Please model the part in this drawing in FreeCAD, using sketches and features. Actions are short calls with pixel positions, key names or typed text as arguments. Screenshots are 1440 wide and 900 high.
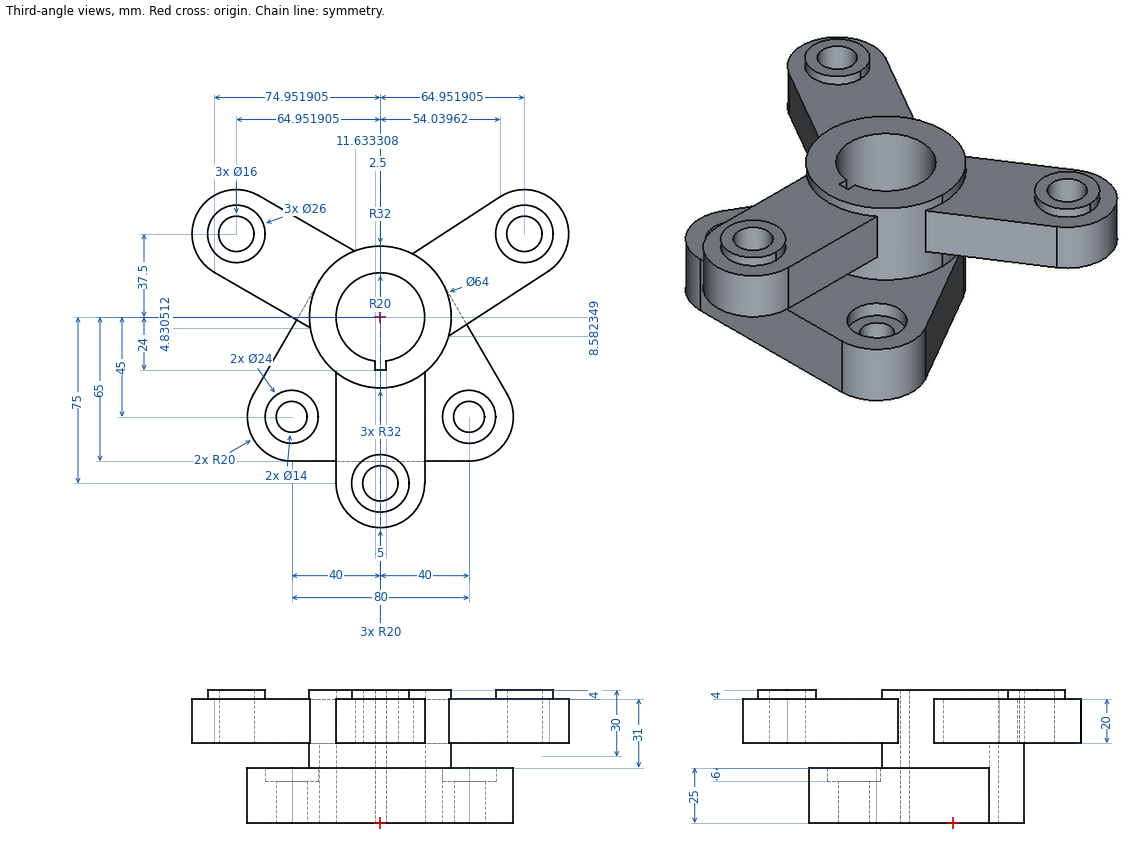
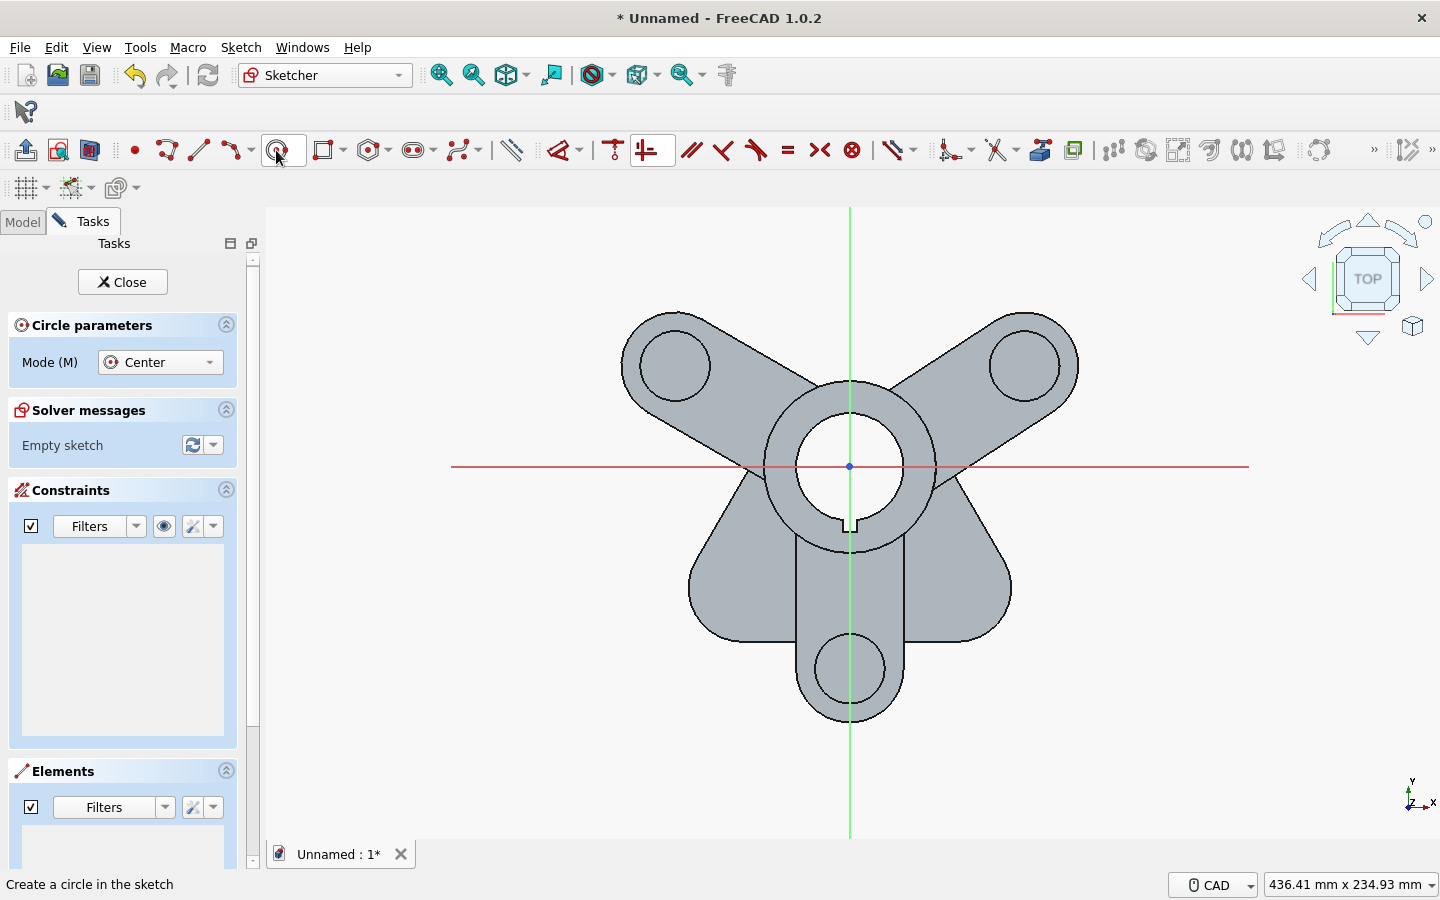
click(675, 366)
move(690, 351)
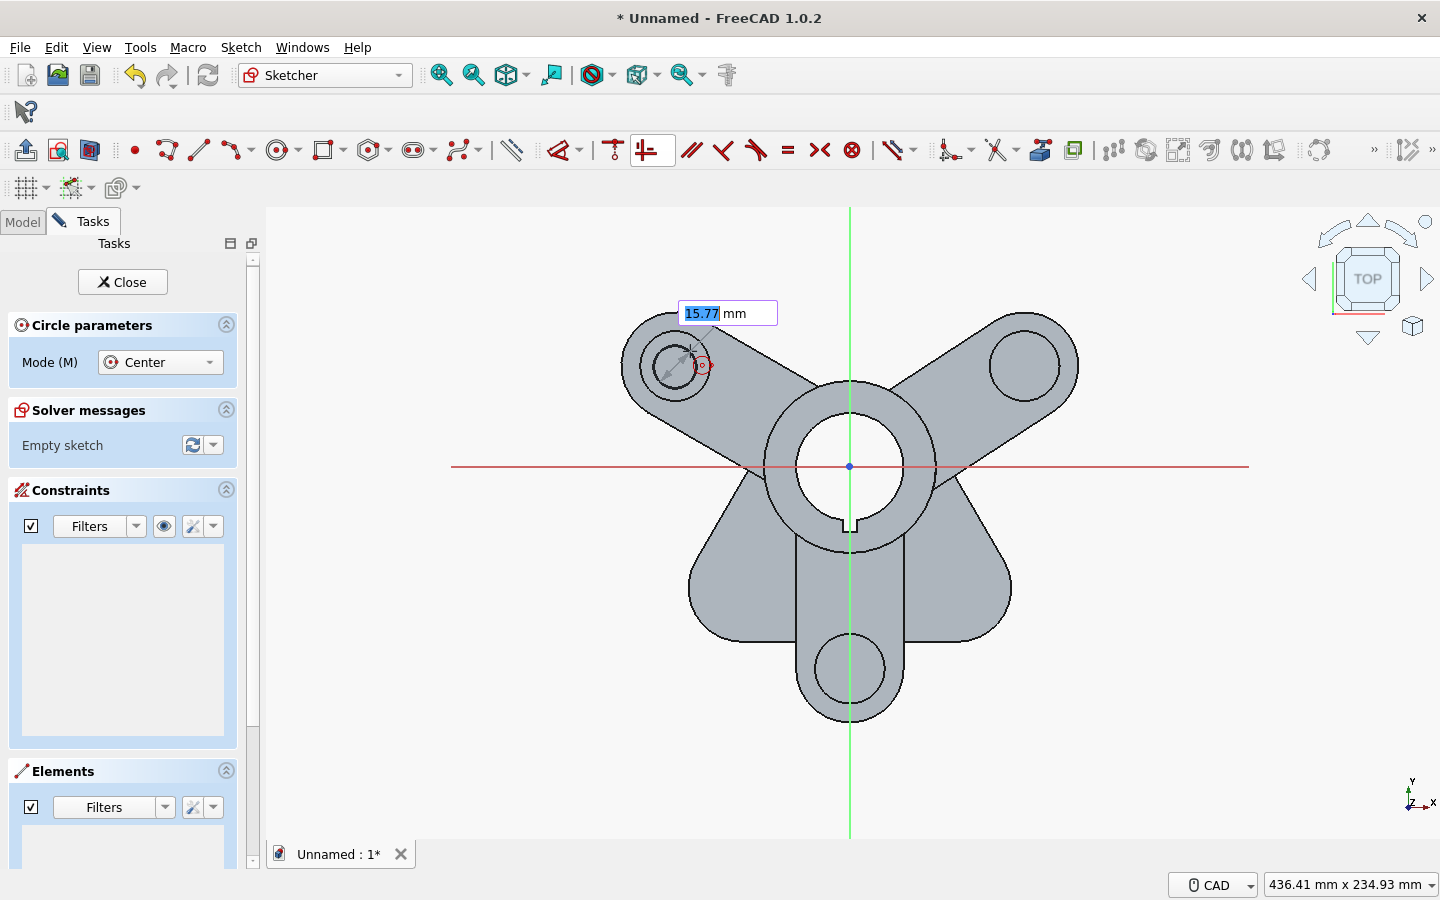
text(16)
key(Return)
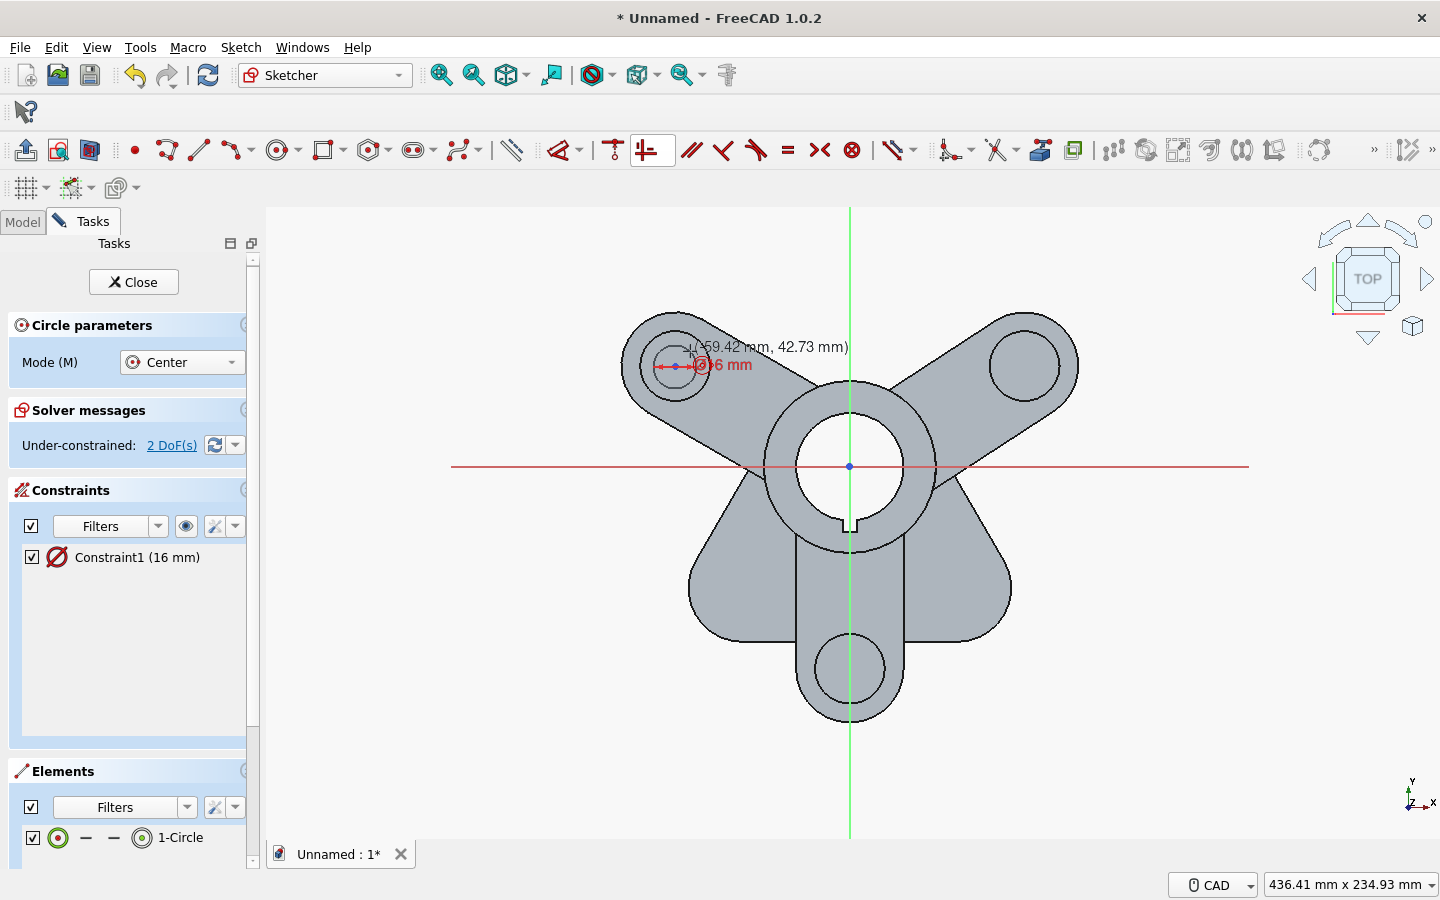
click(1025, 366)
move(1040, 351)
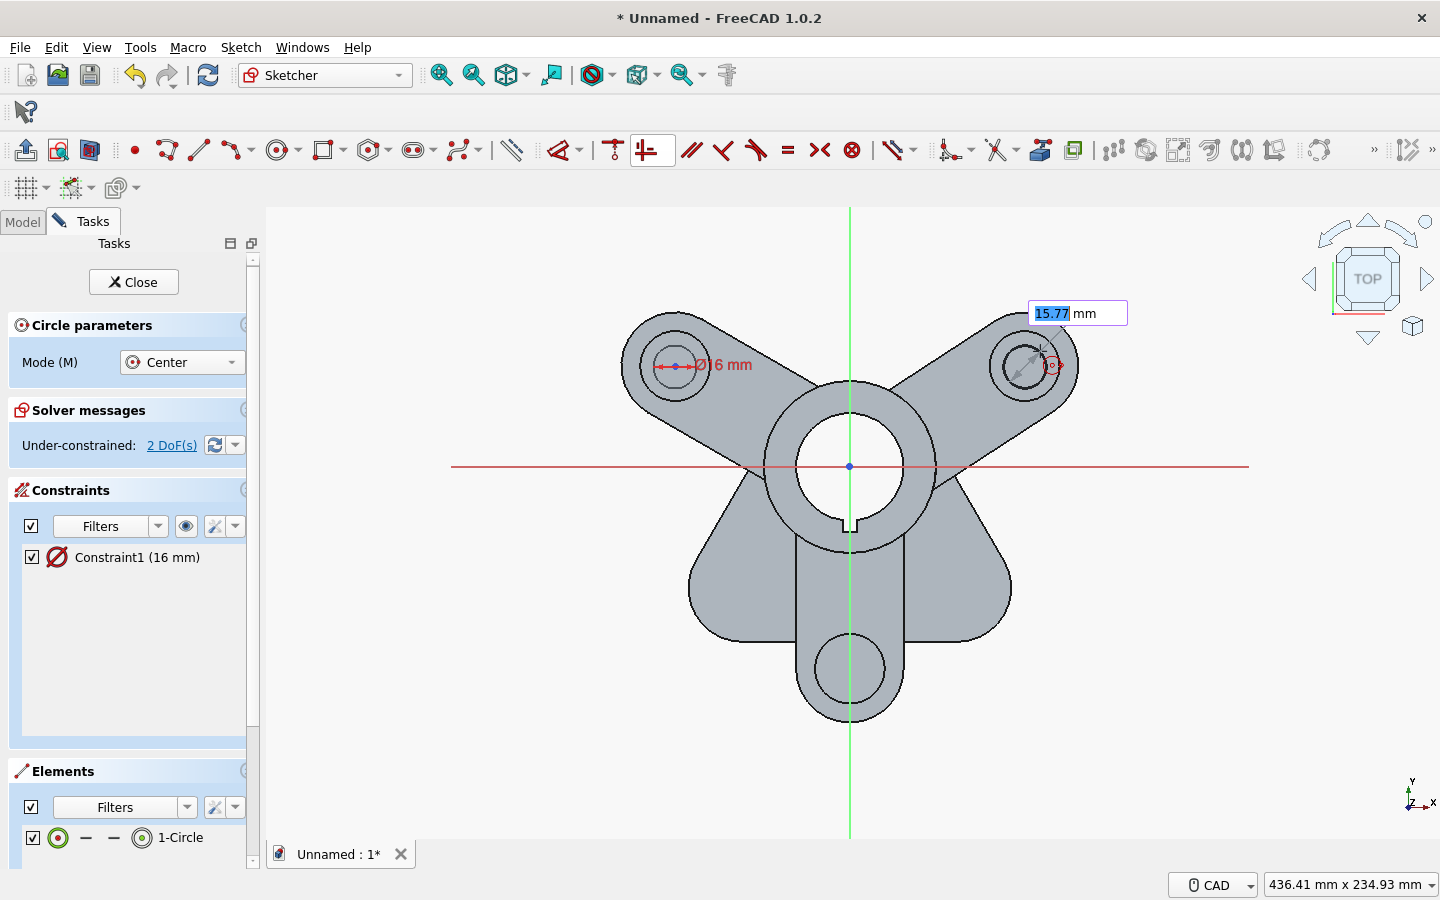
text(16)
key(Return)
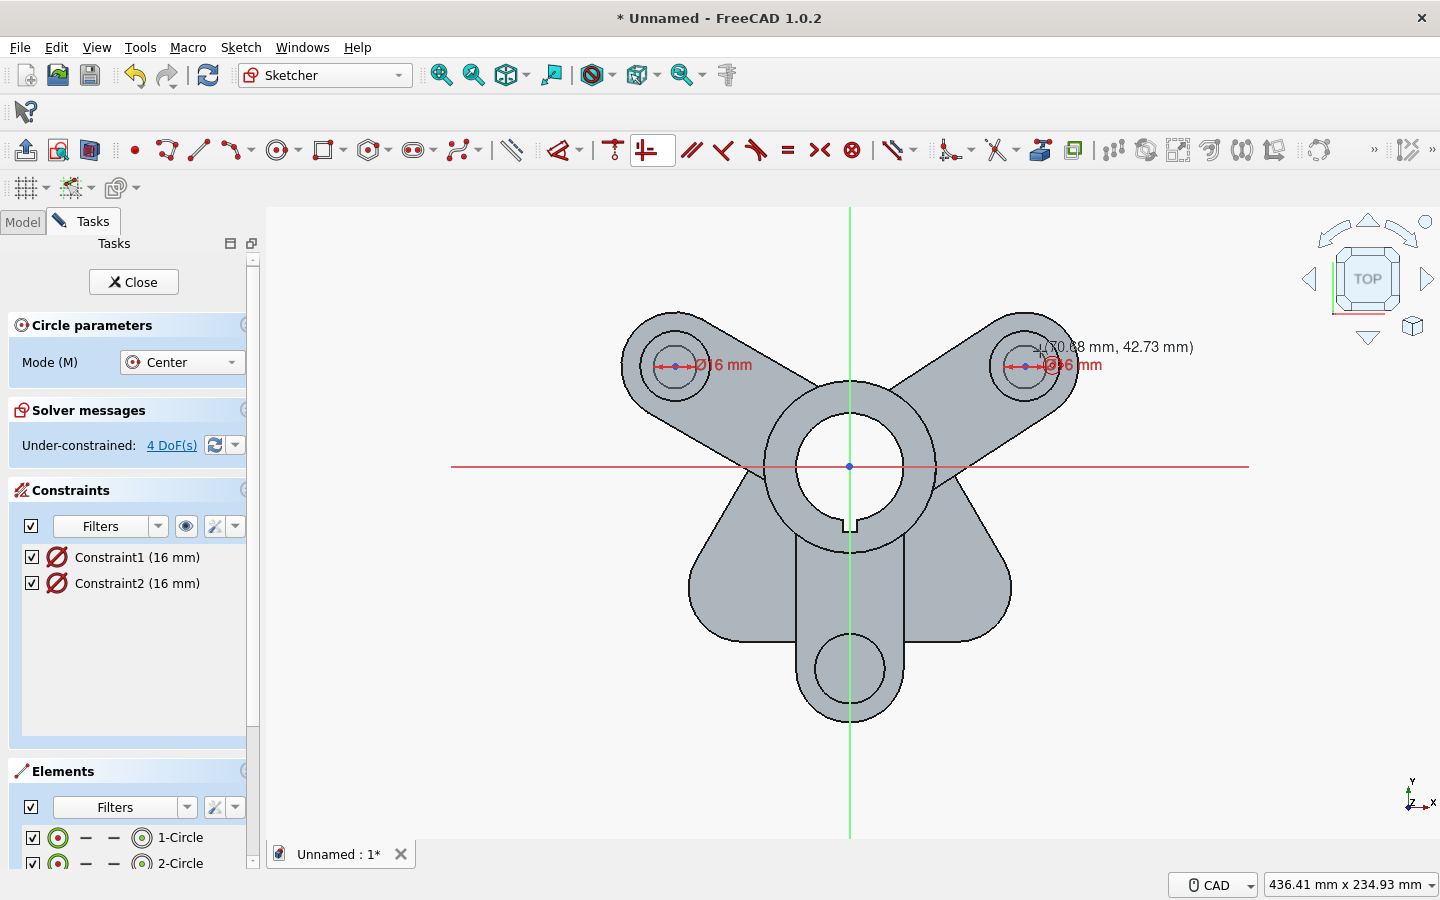
click(850, 669)
move(865, 654)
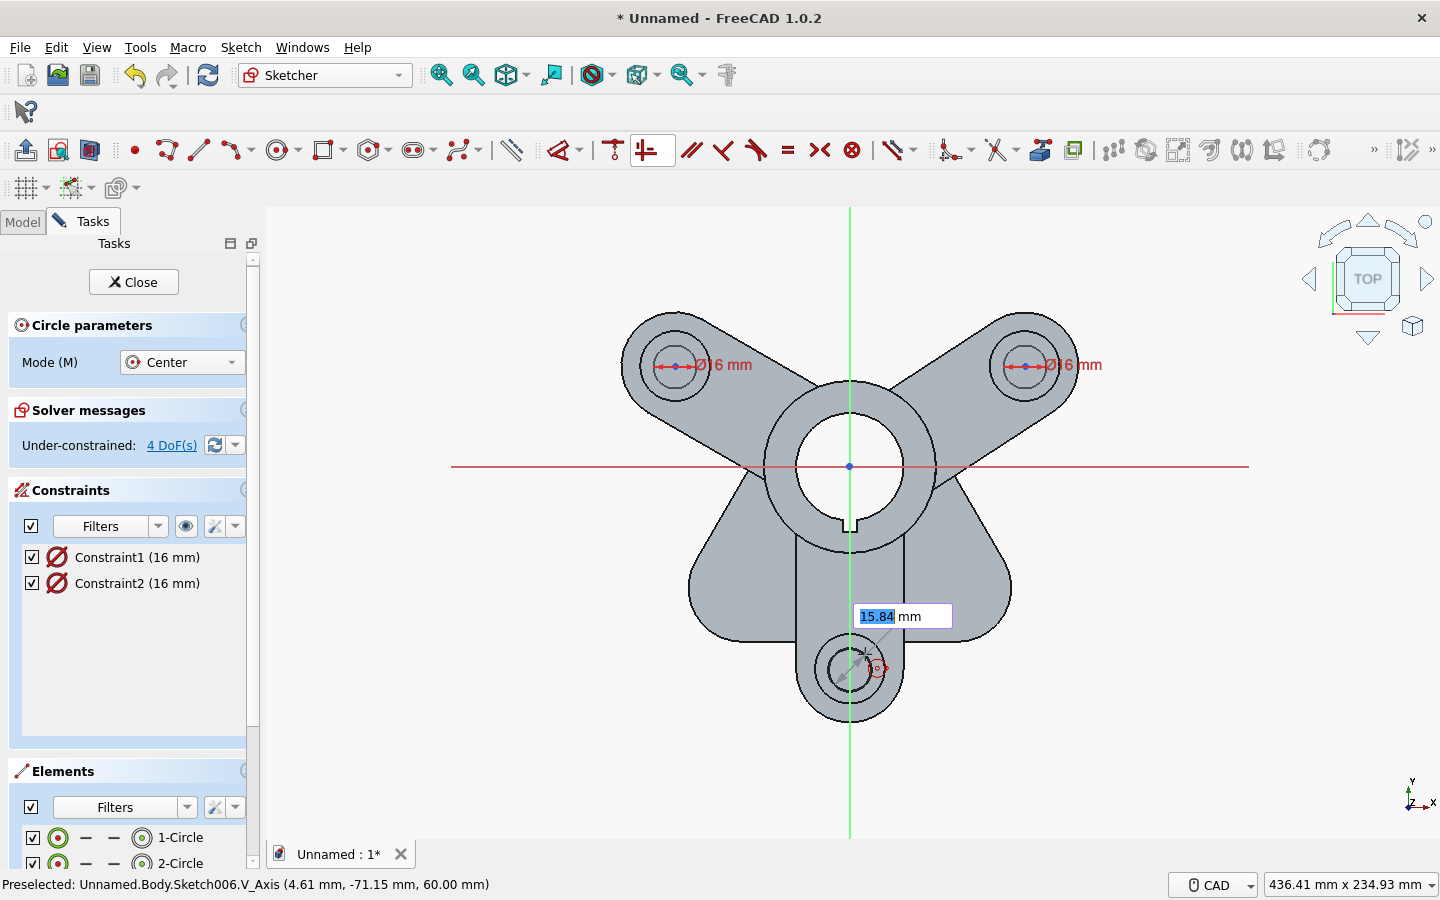
text(16)
key(Return)
key(Escape)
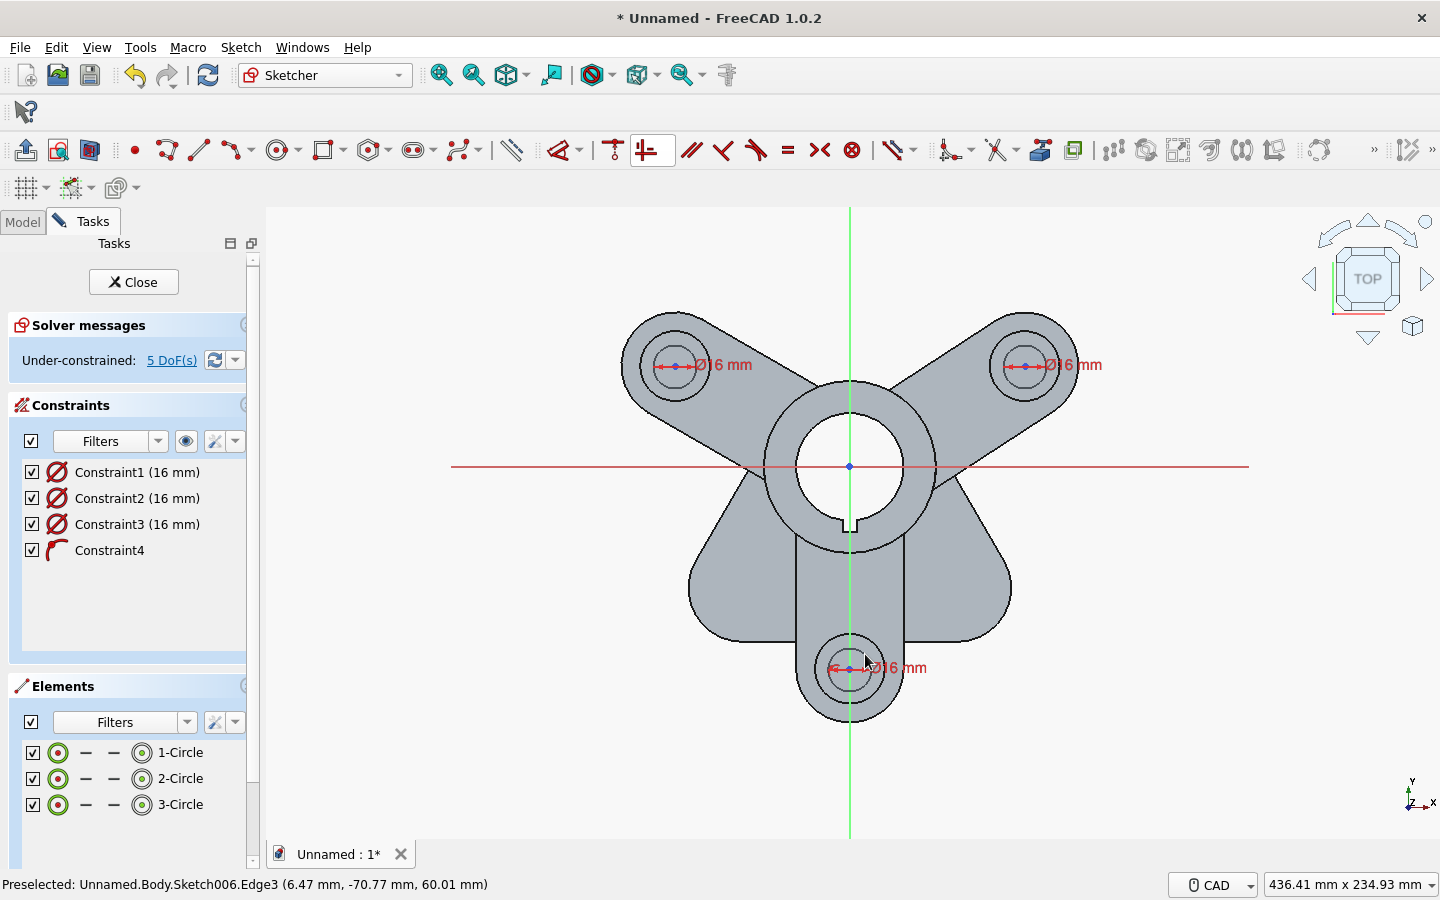
click(675, 367)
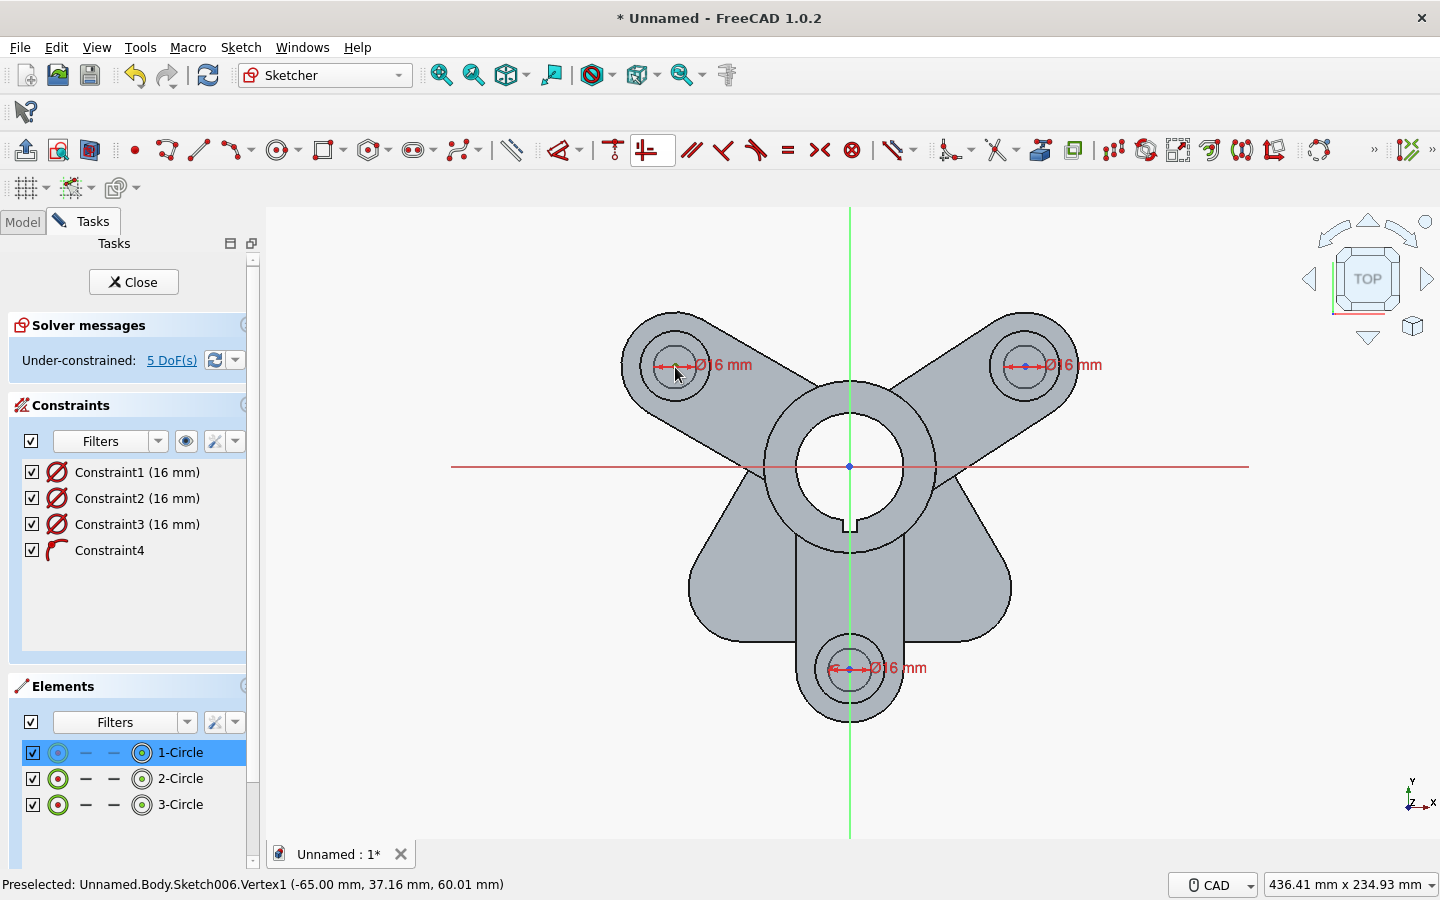
click(1025, 367)